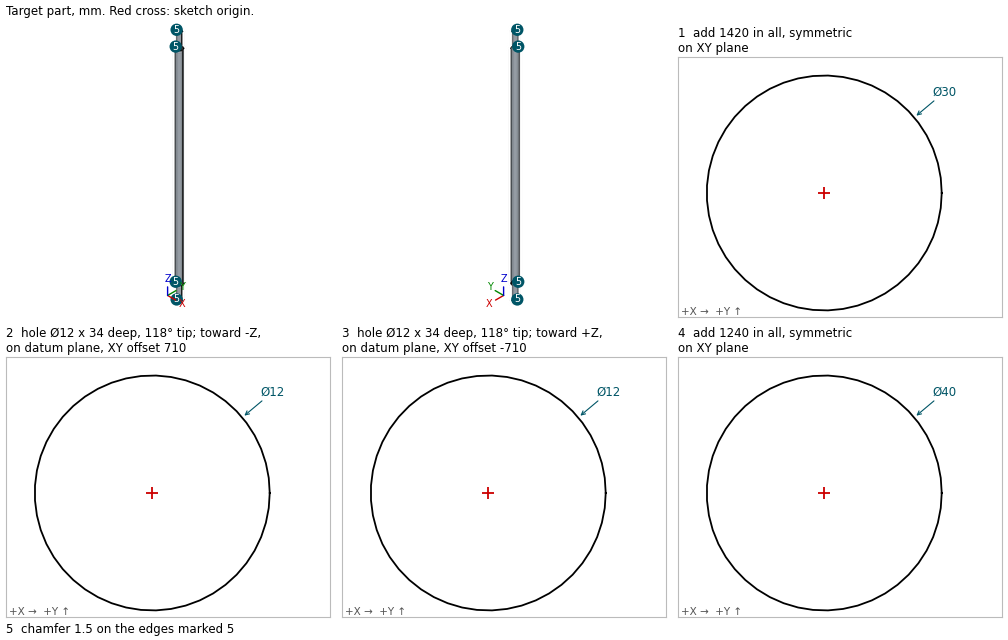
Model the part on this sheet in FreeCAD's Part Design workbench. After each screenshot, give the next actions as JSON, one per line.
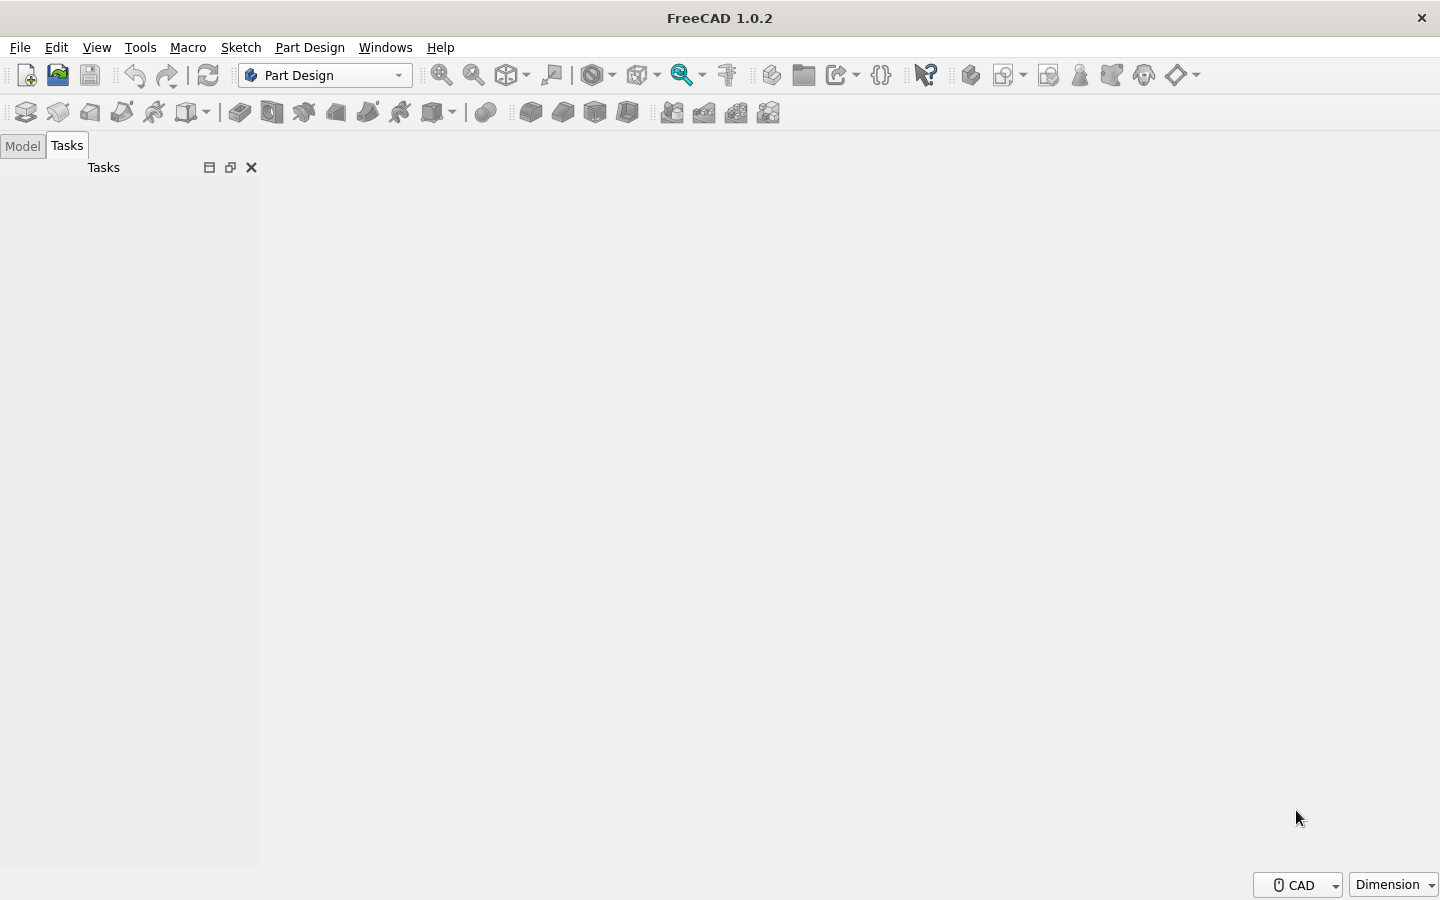
{"action": "left_click", "coordinate": [26, 76]}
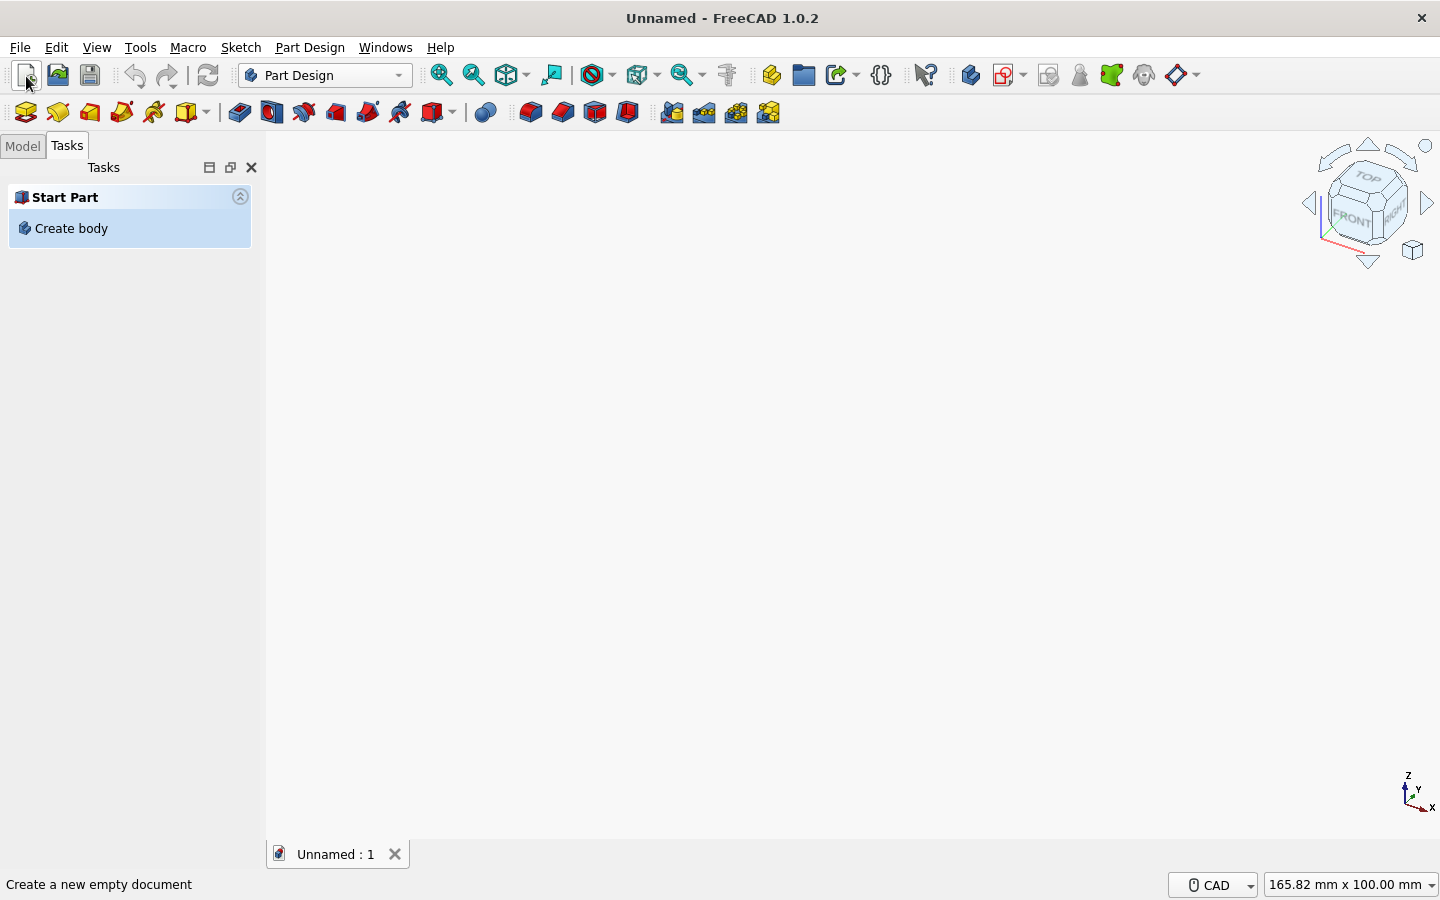
{"action": "left_click", "coordinate": [1004, 76]}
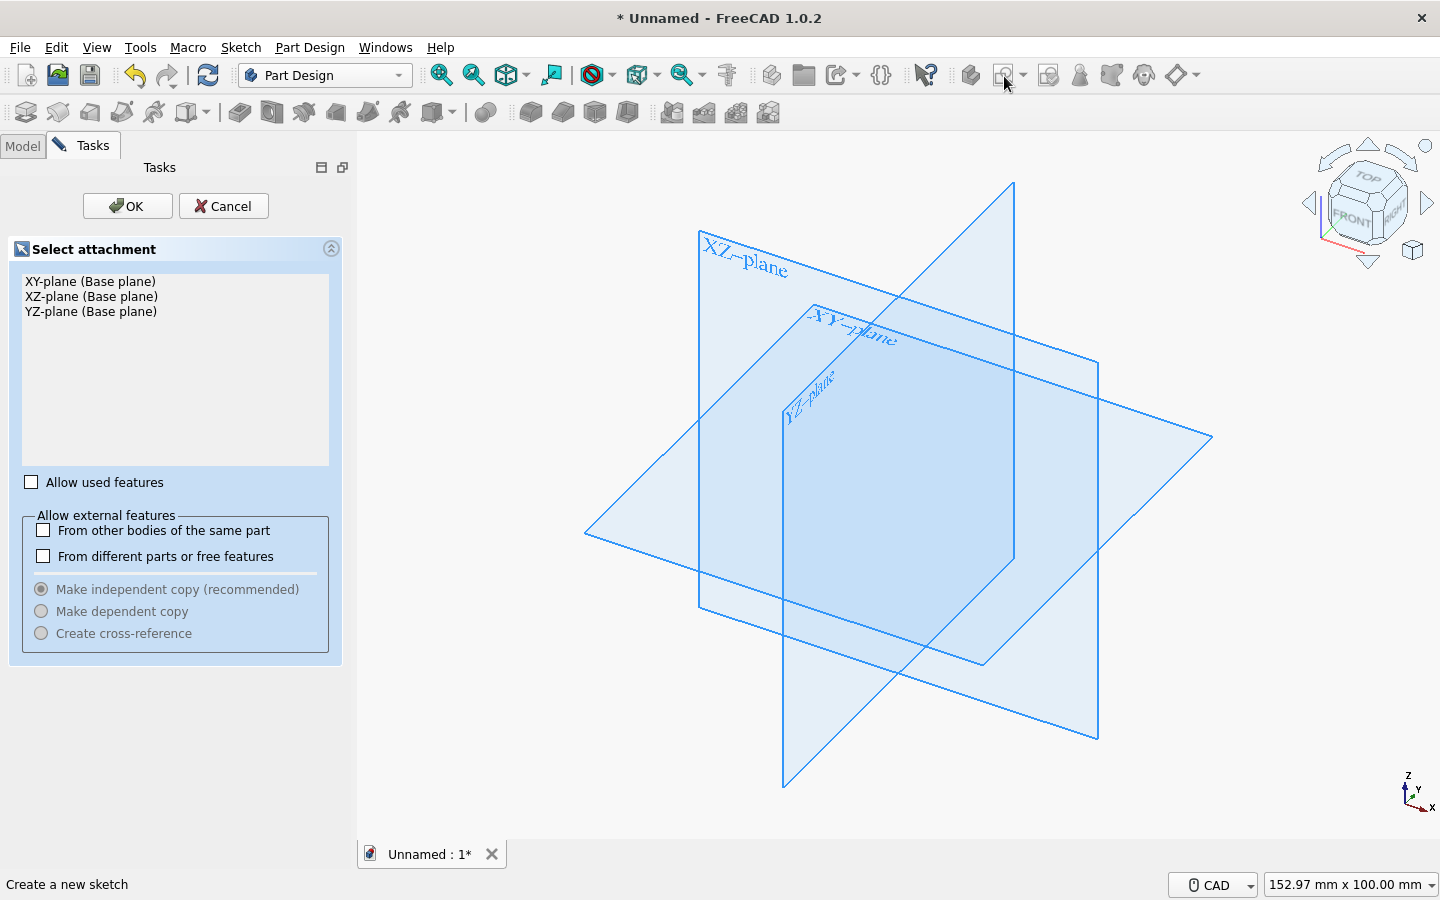
{"action": "left_click", "coordinate": [82, 282]}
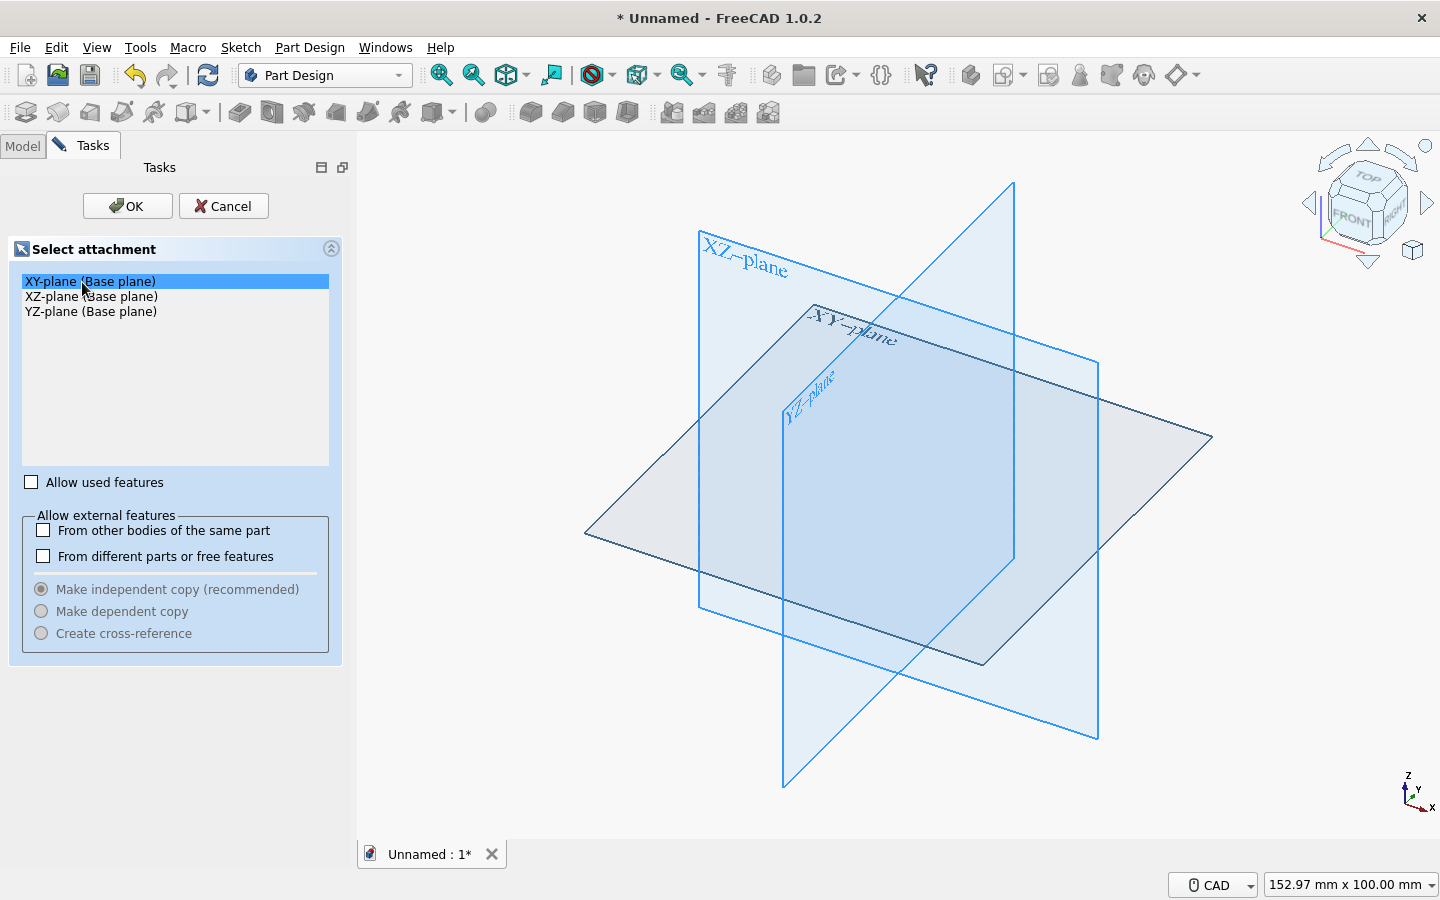
{"action": "left_click", "coordinate": [128, 206]}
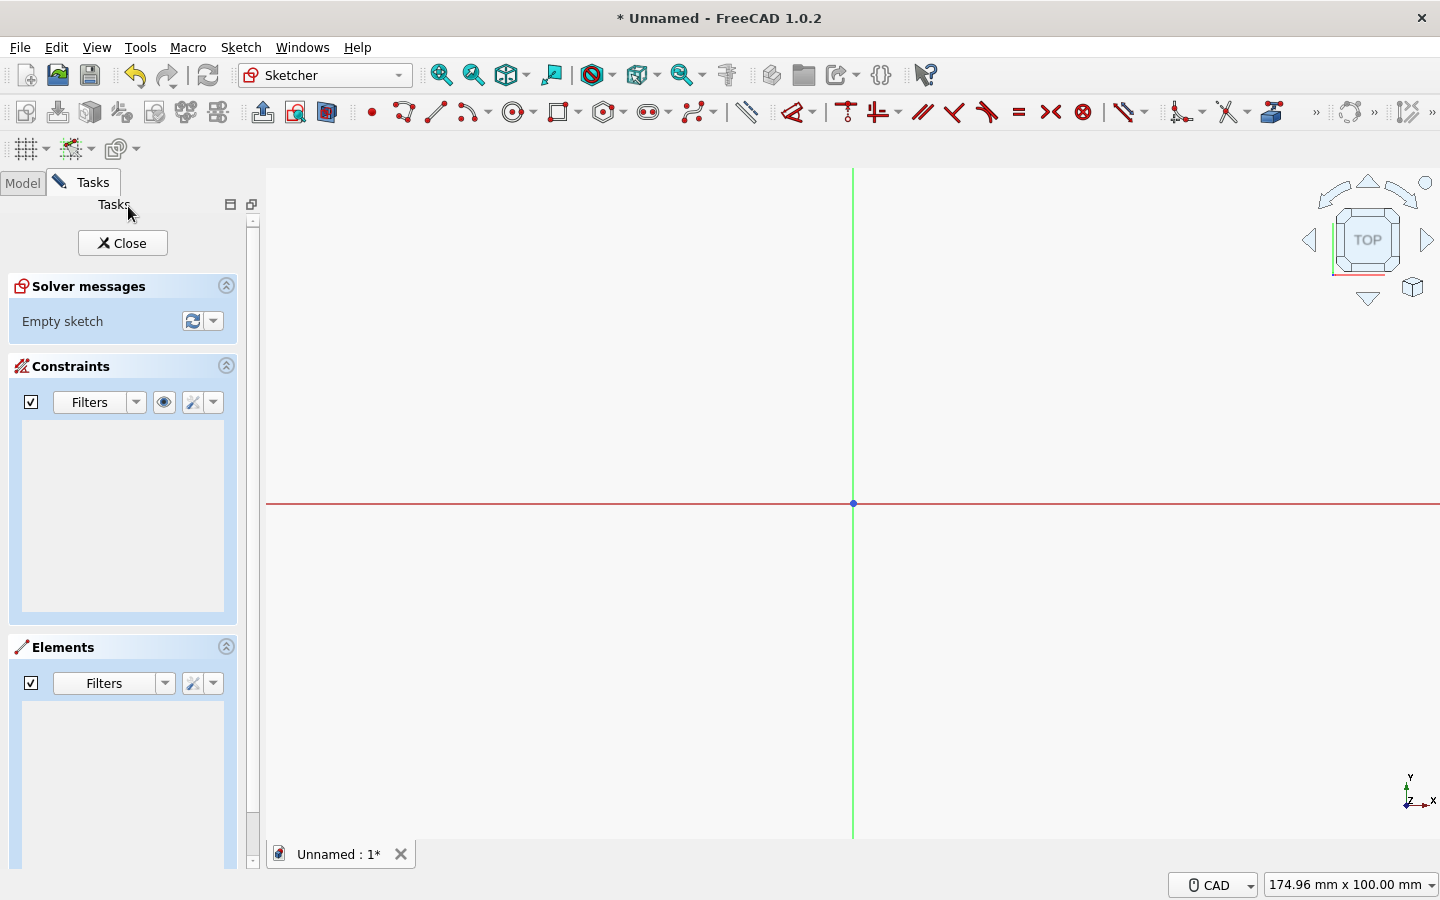
{"action": "scroll", "coordinate": [909, 504], "scroll_direction": "up", "scroll_amount": 4}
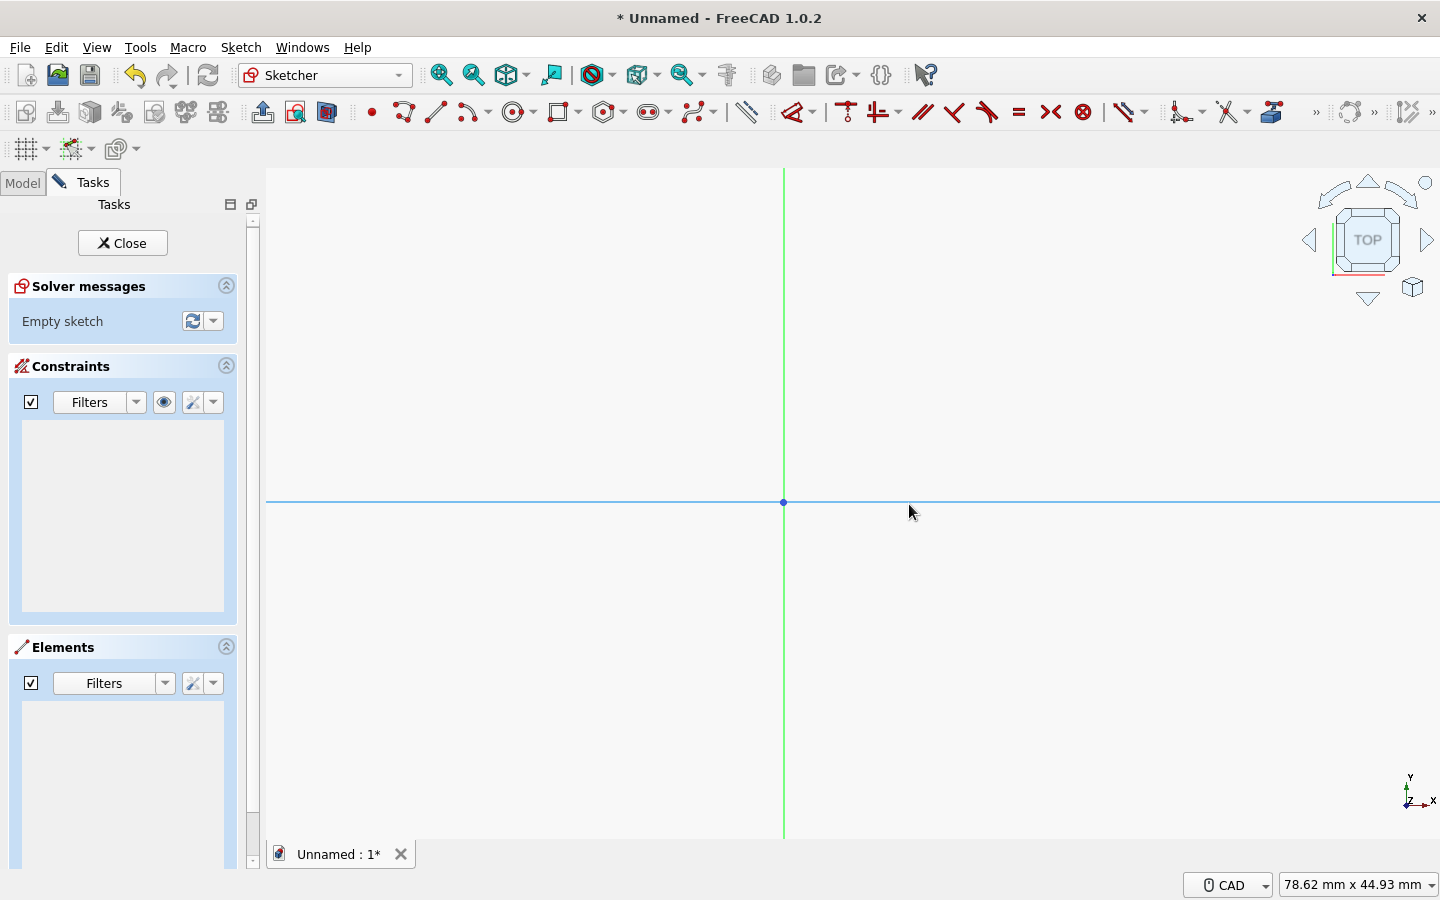
{"action": "left_click", "coordinate": [514, 112]}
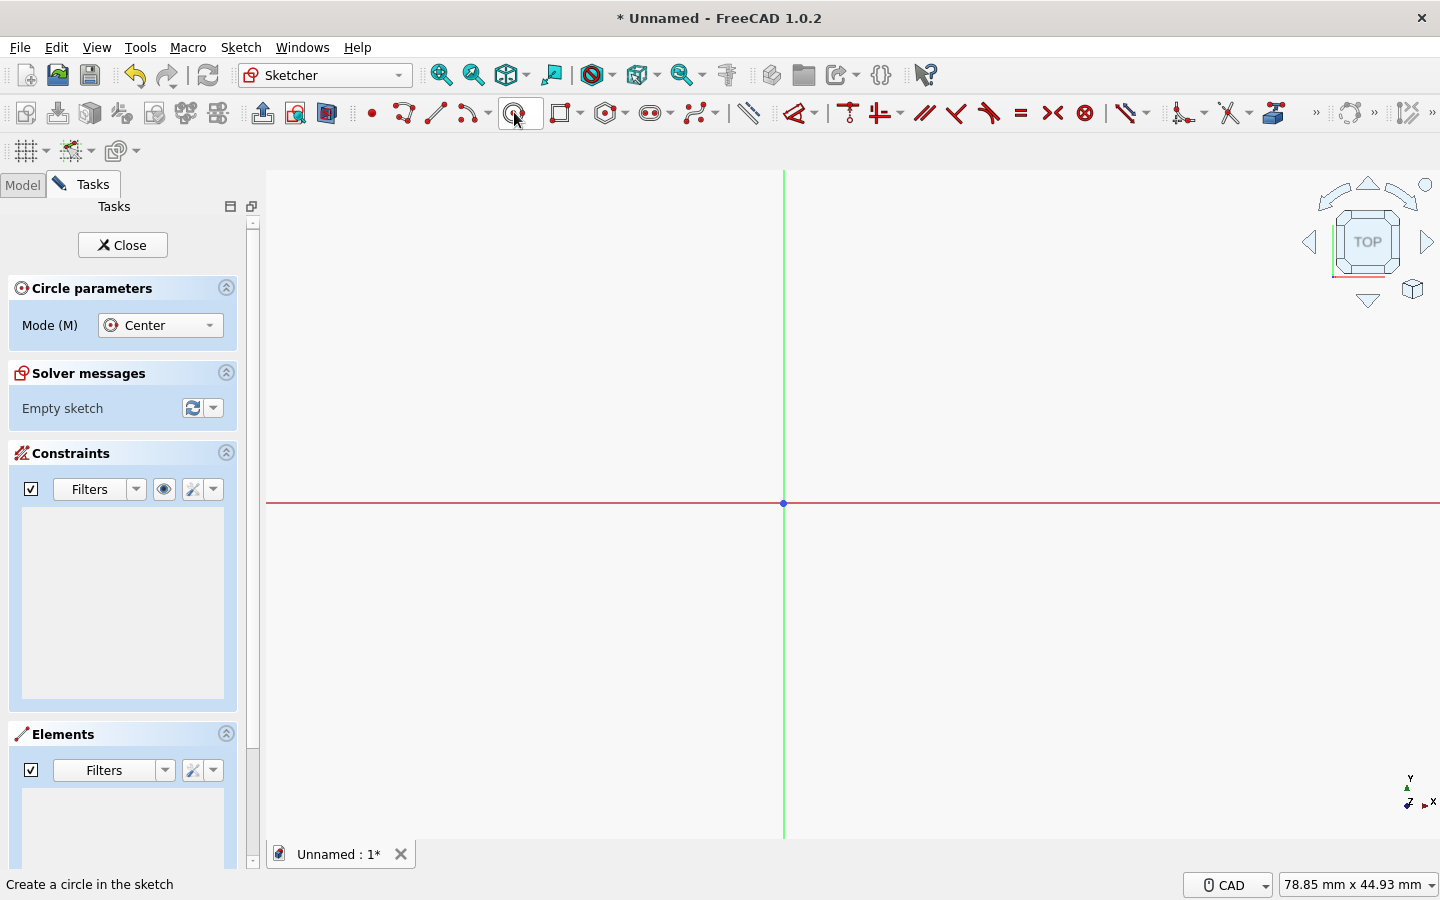
{"action": "left_click", "coordinate": [784, 503]}
{"action": "mouse_move", "coordinate": [942, 345]}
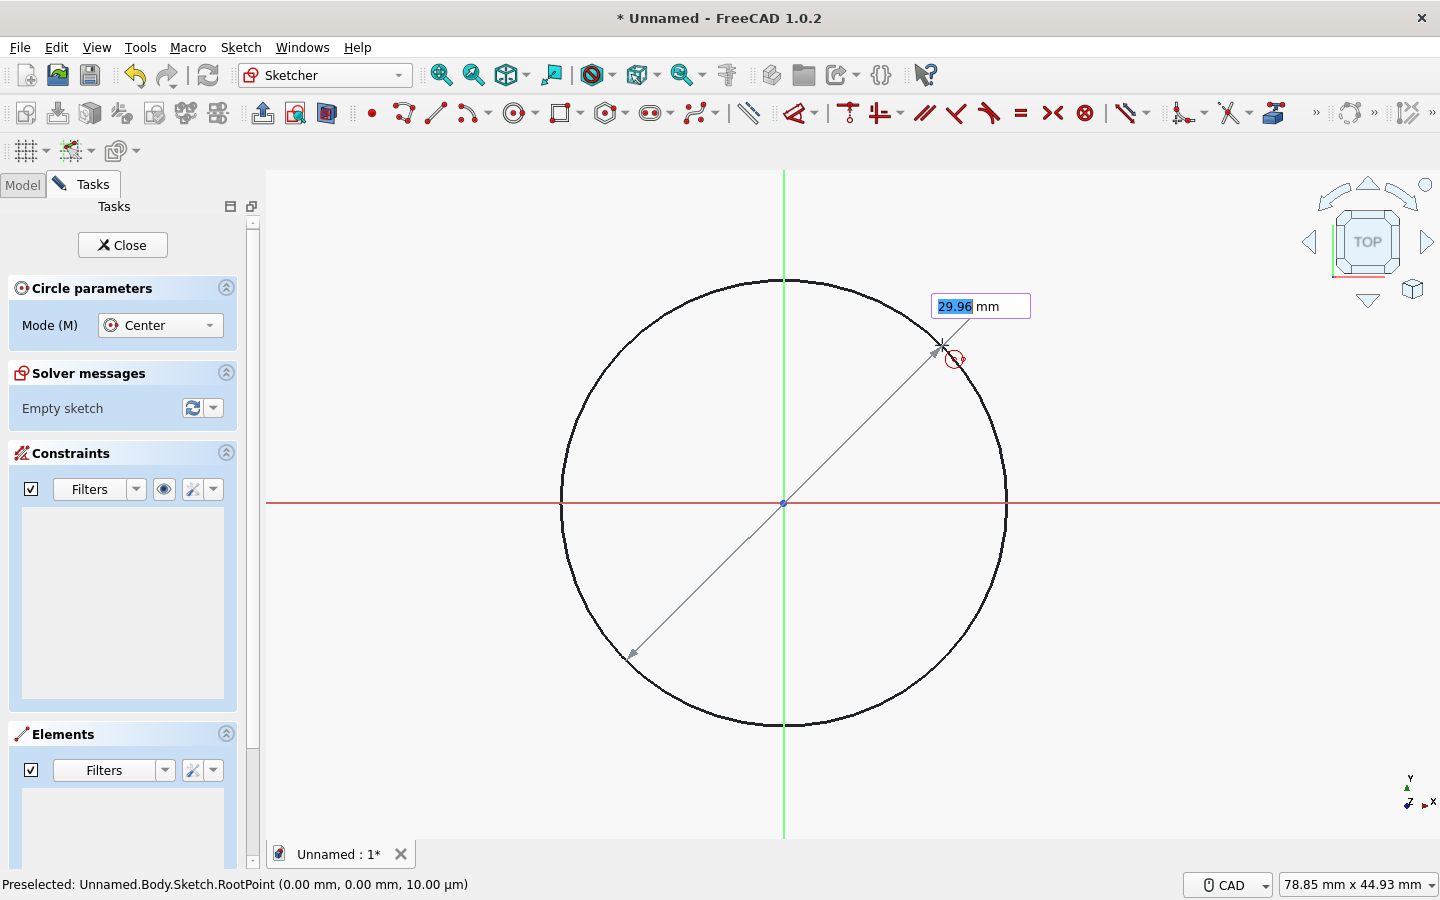
{"action": "type", "text": "30"}
{"action": "key", "text": "Return"}
{"action": "key", "text": "Escape"}